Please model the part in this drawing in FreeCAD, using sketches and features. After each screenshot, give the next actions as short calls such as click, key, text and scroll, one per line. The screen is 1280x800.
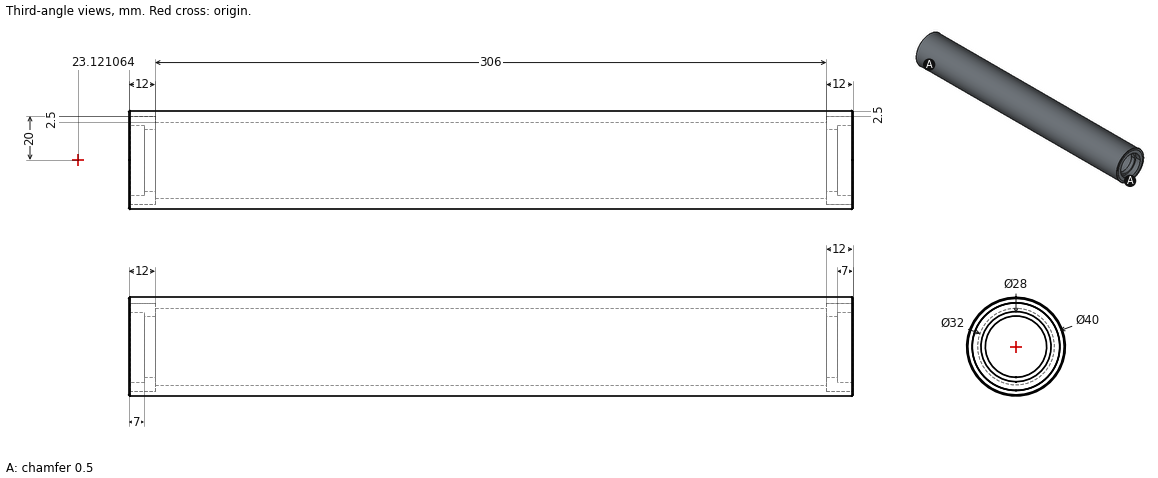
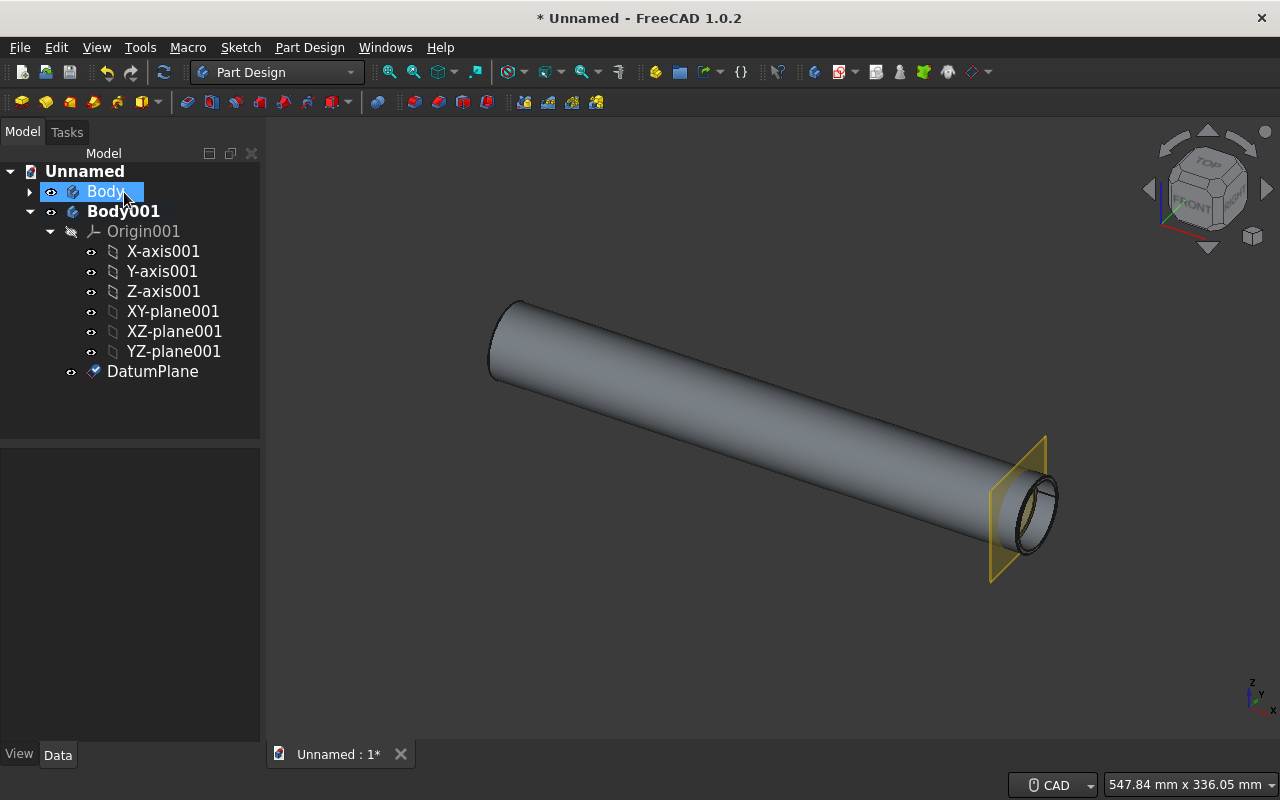
click(116, 372)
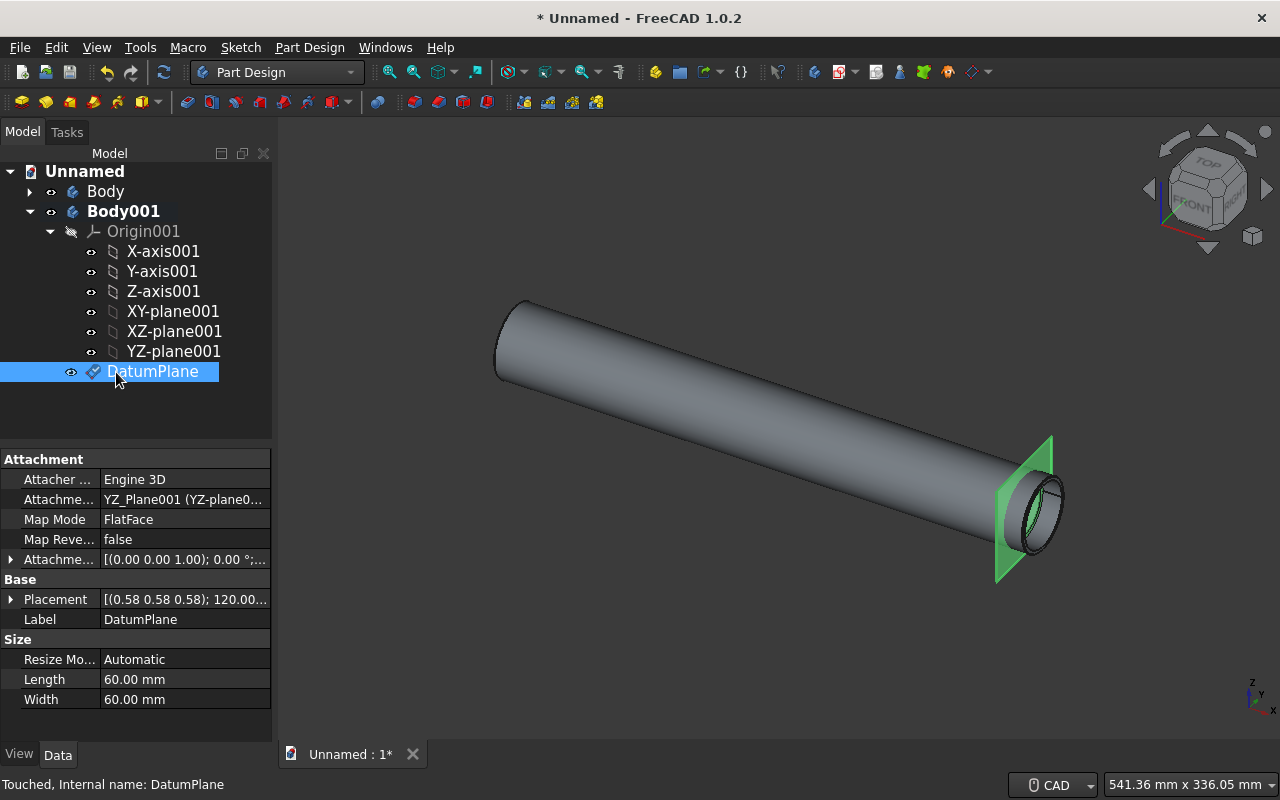
click(840, 72)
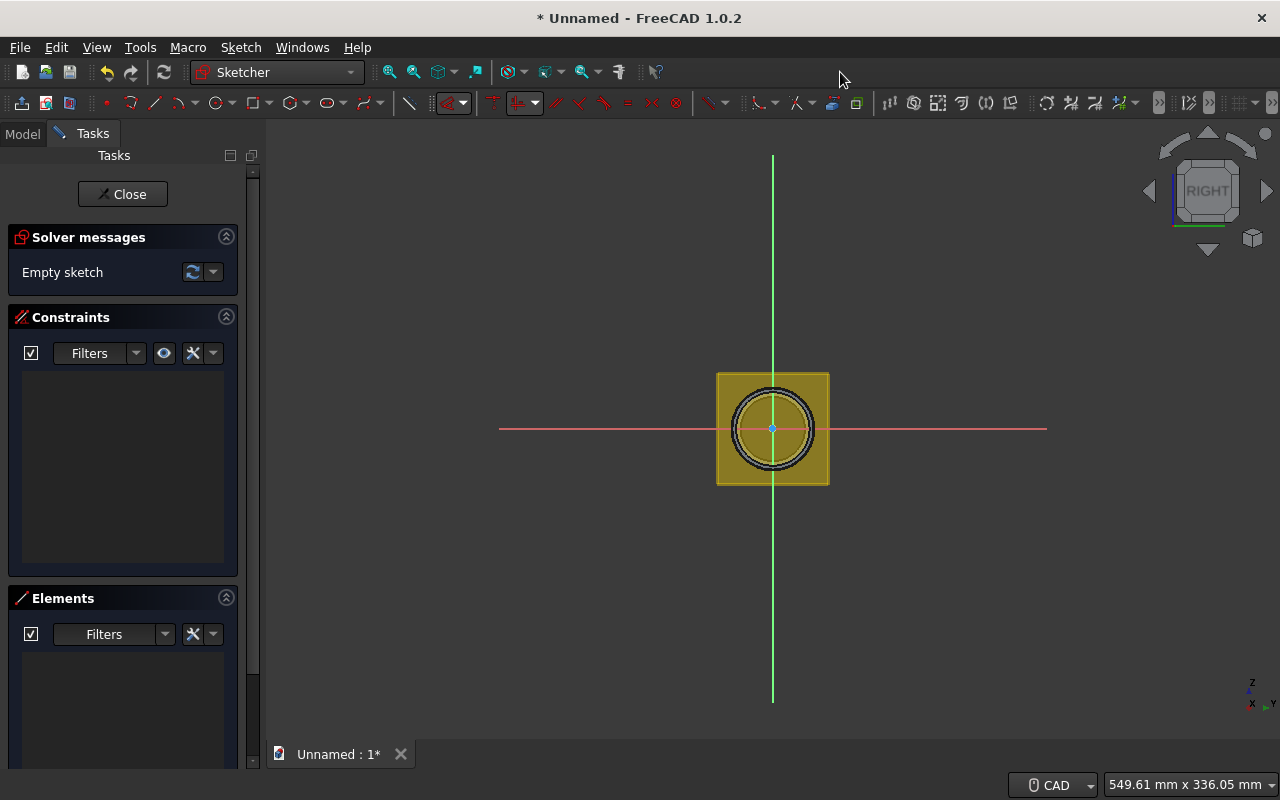
scroll(790, 429, up, 8)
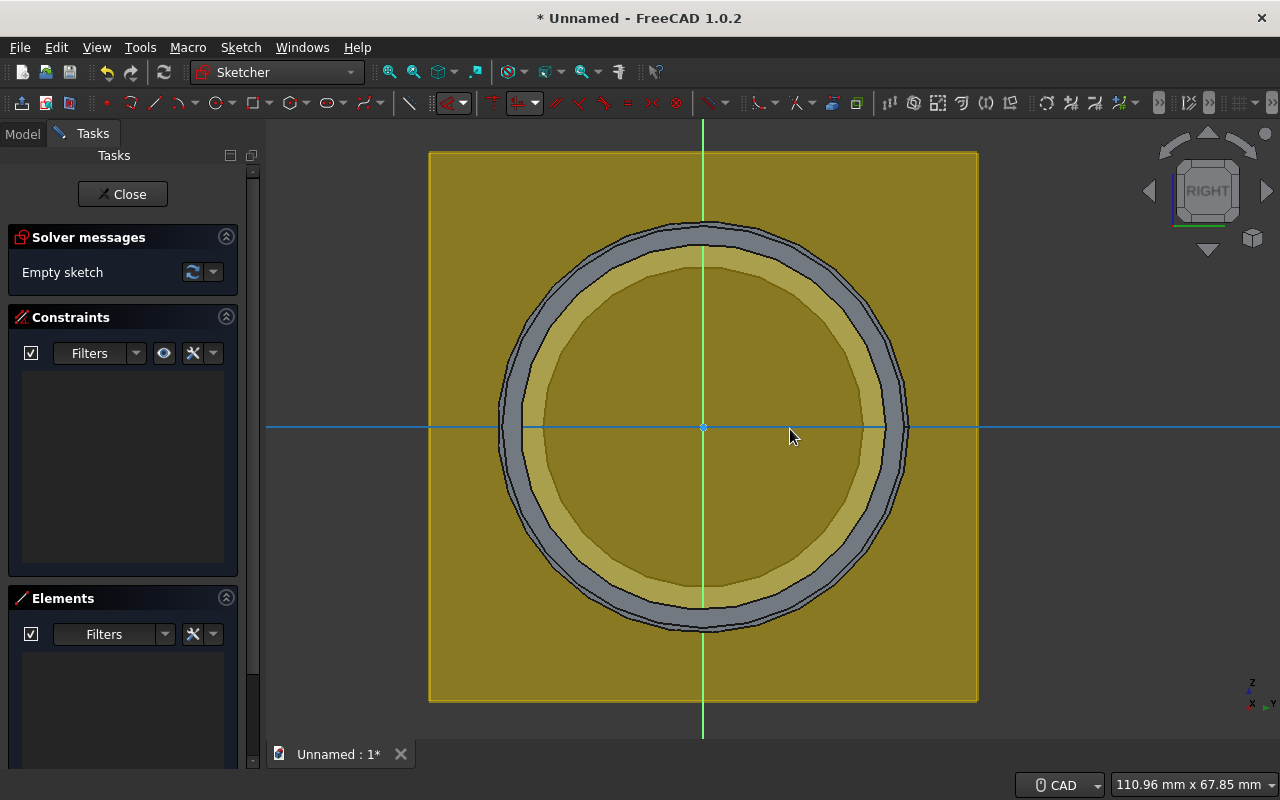
click(216, 104)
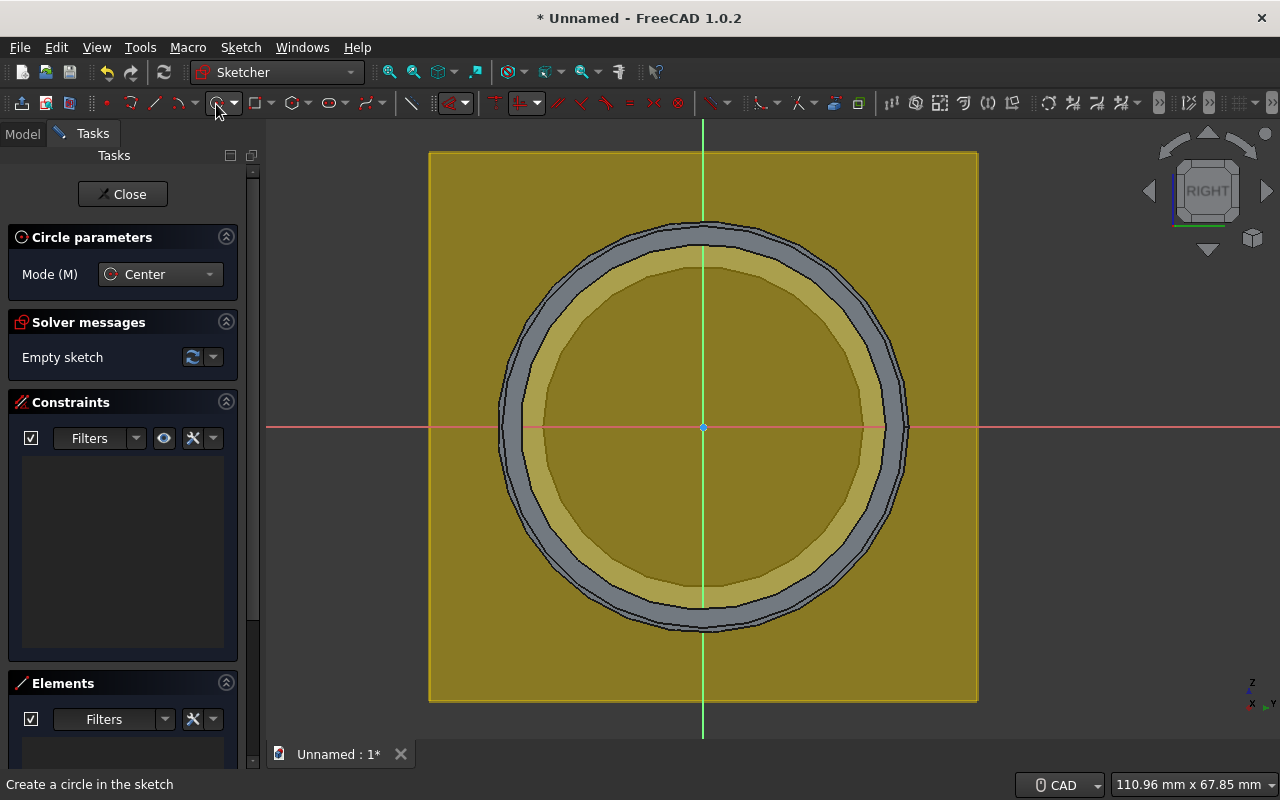
click(703, 427)
move(832, 298)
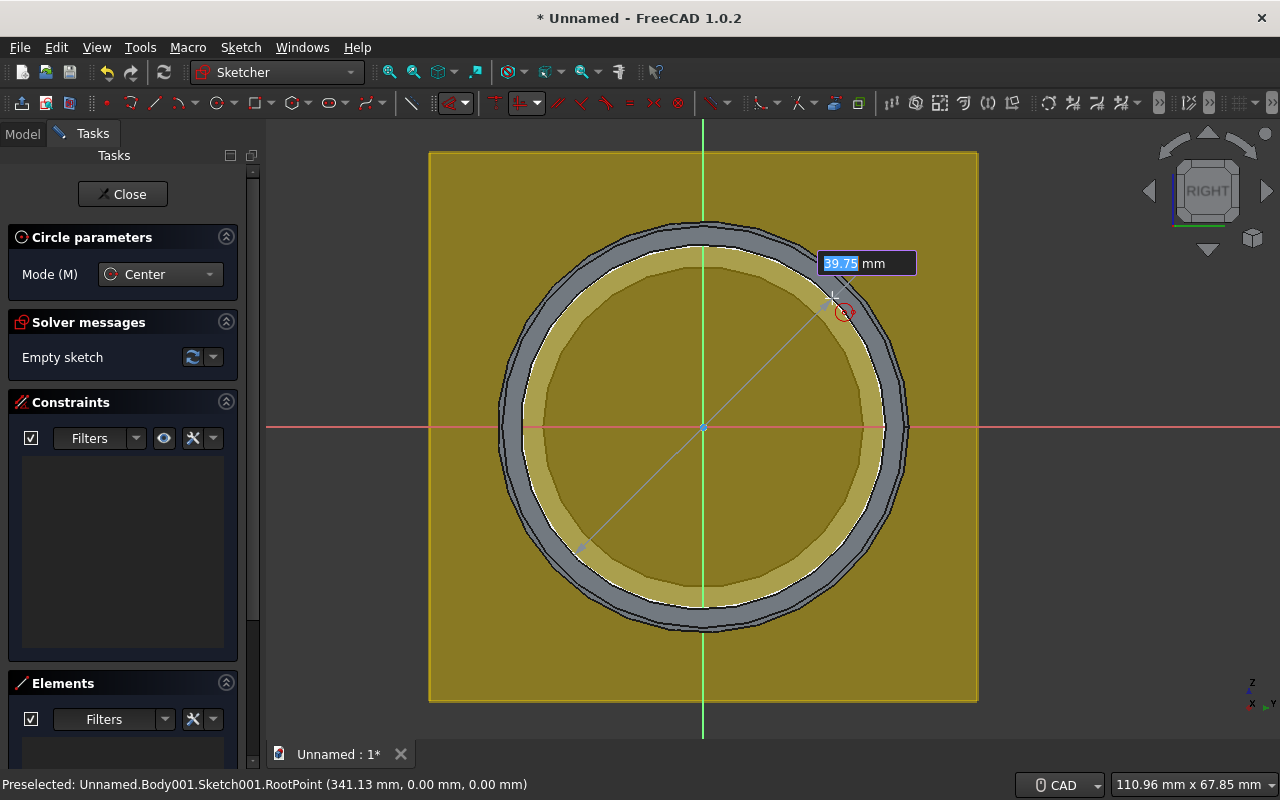
text(40)
key(Return)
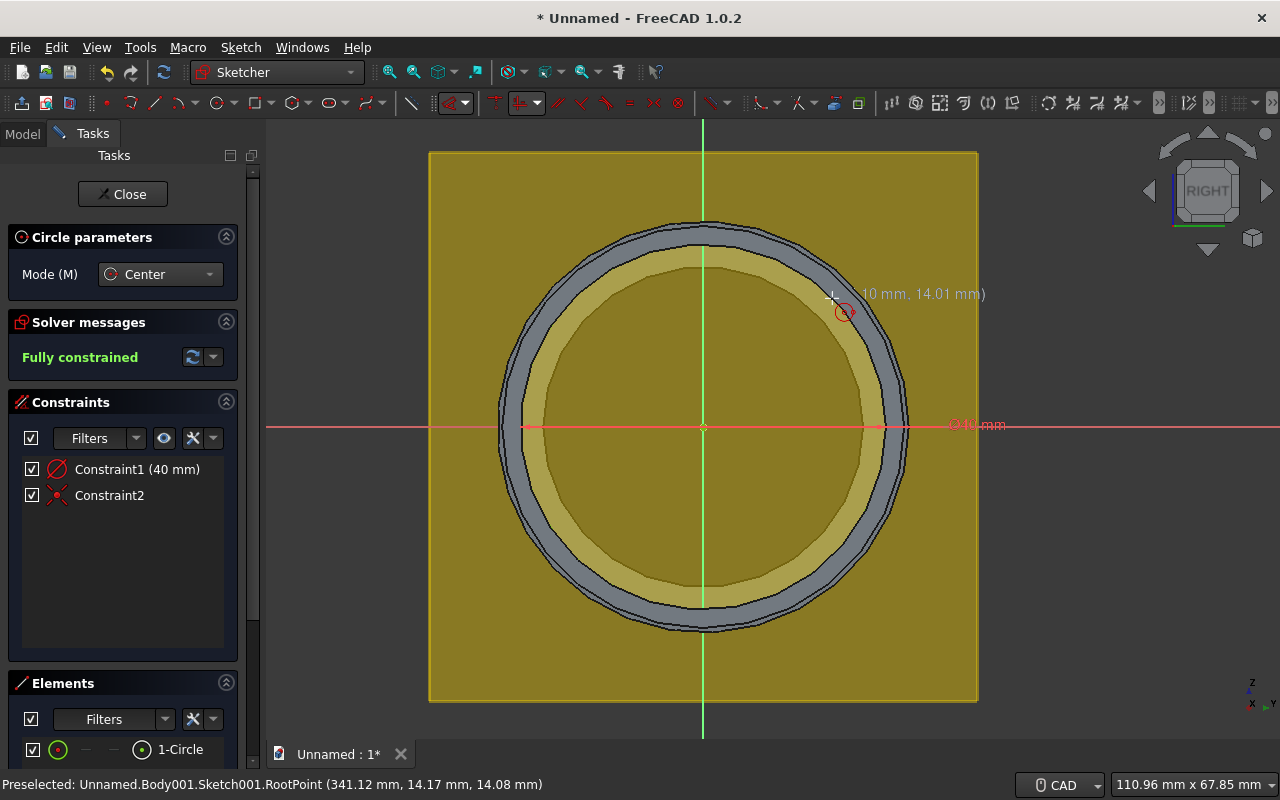
click(703, 427)
move(794, 337)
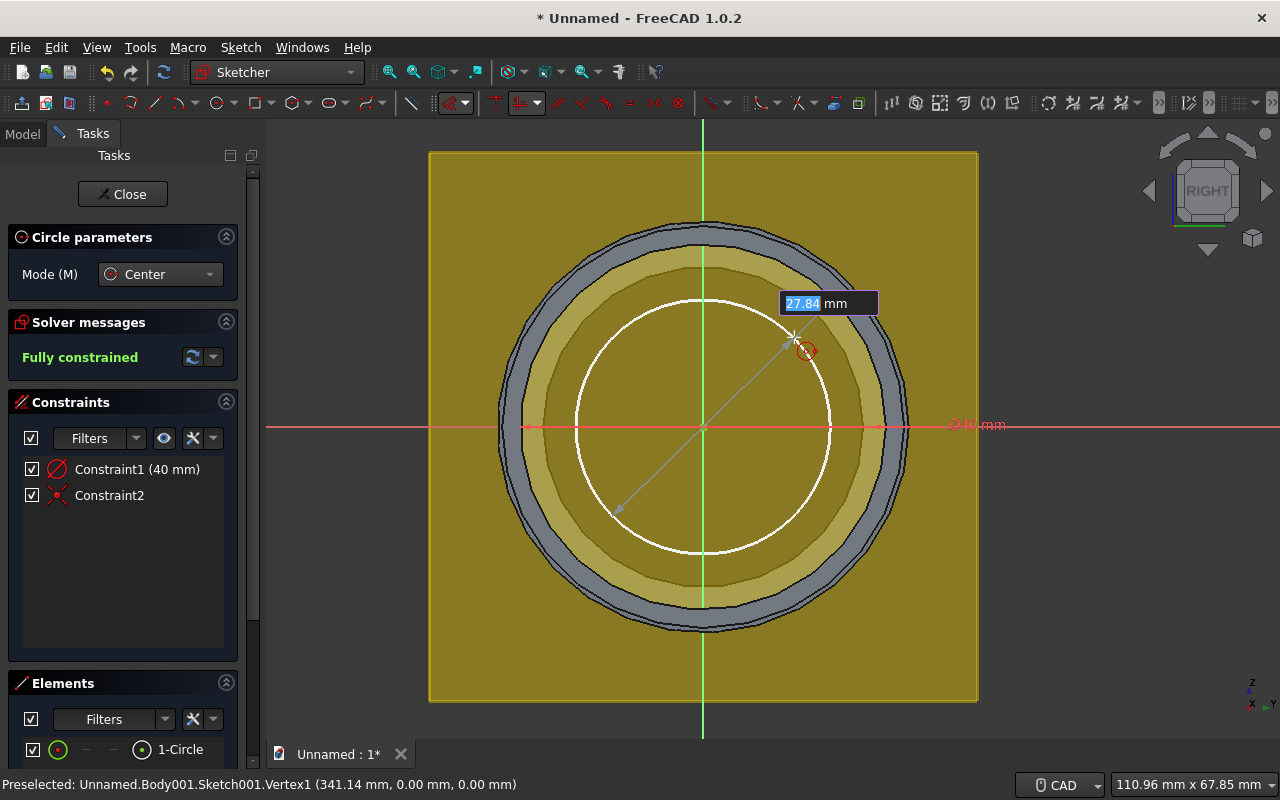
text(28)
key(Return)
key(Escape)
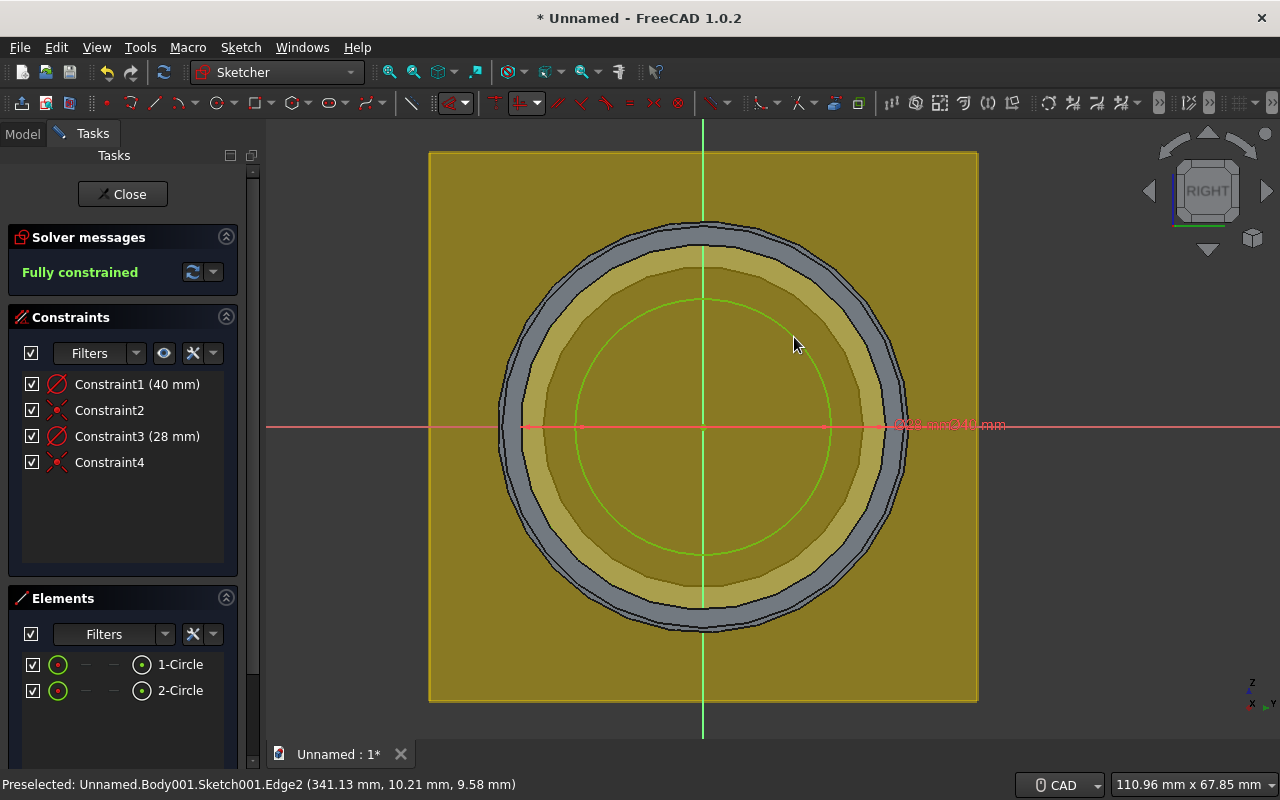
click(123, 194)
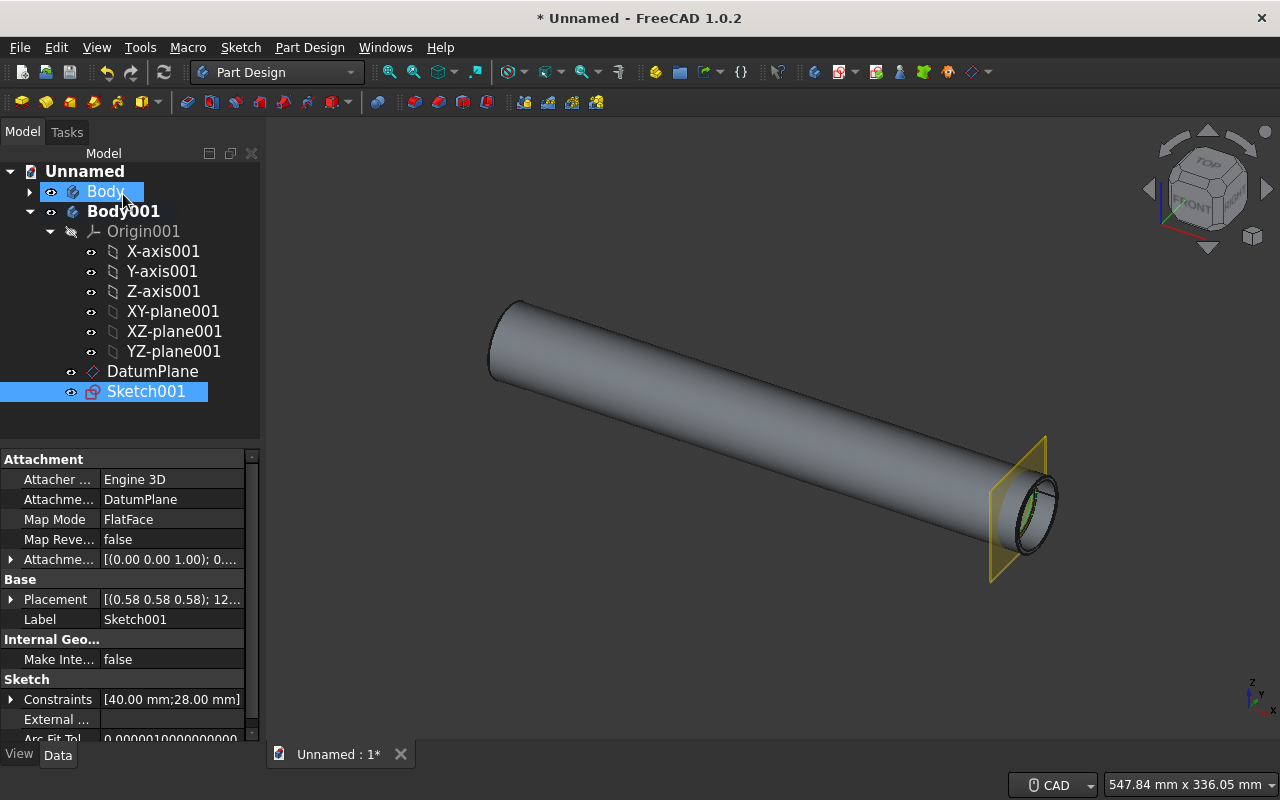
click(22, 102)